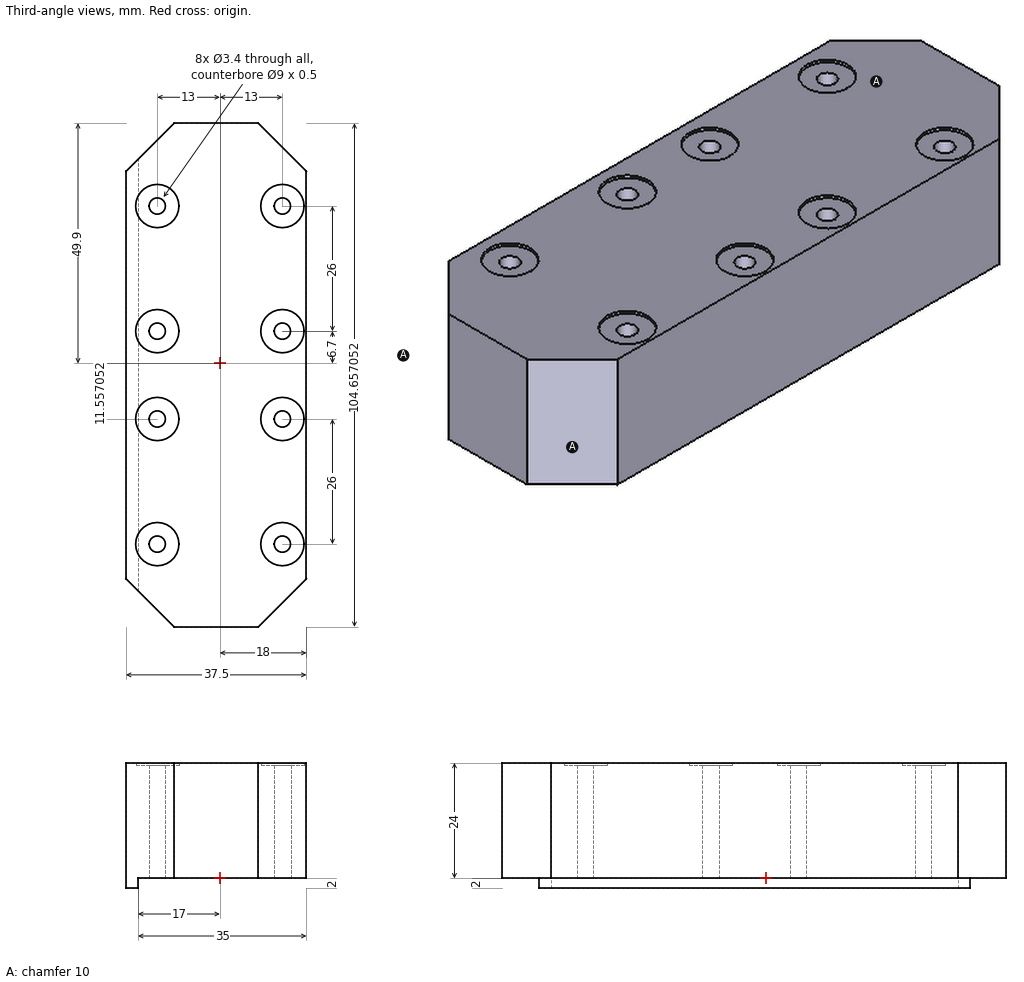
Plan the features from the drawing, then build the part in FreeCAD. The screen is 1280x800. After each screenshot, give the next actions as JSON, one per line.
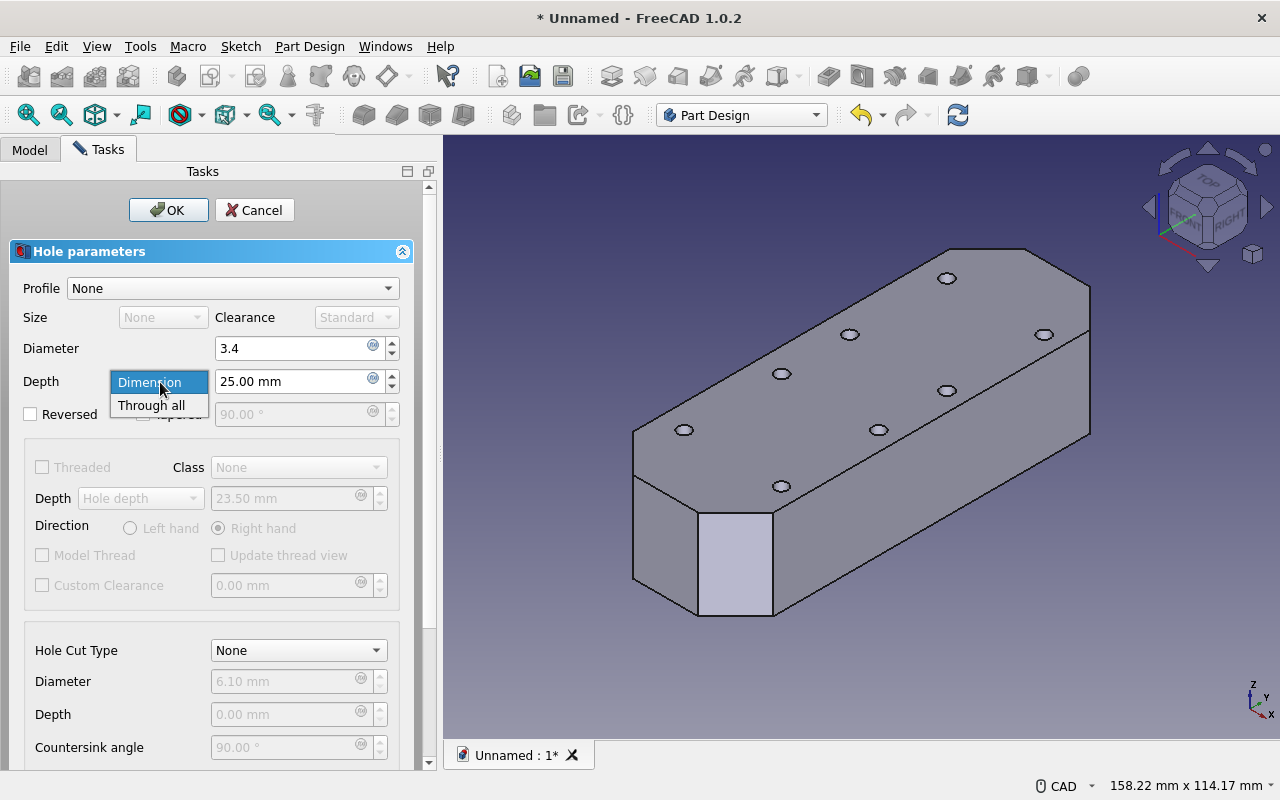
{"action": "left_click", "coordinate": [158, 406]}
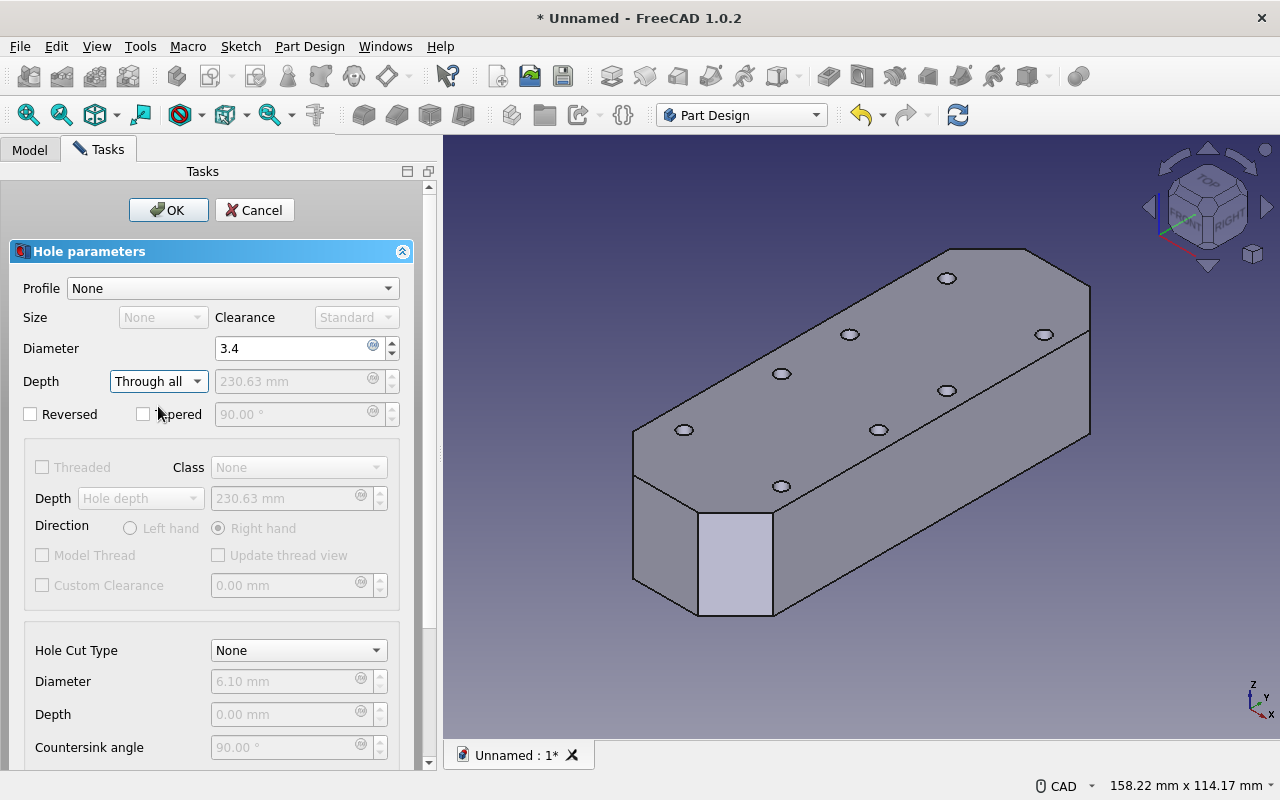
{"action": "left_click", "coordinate": [300, 650]}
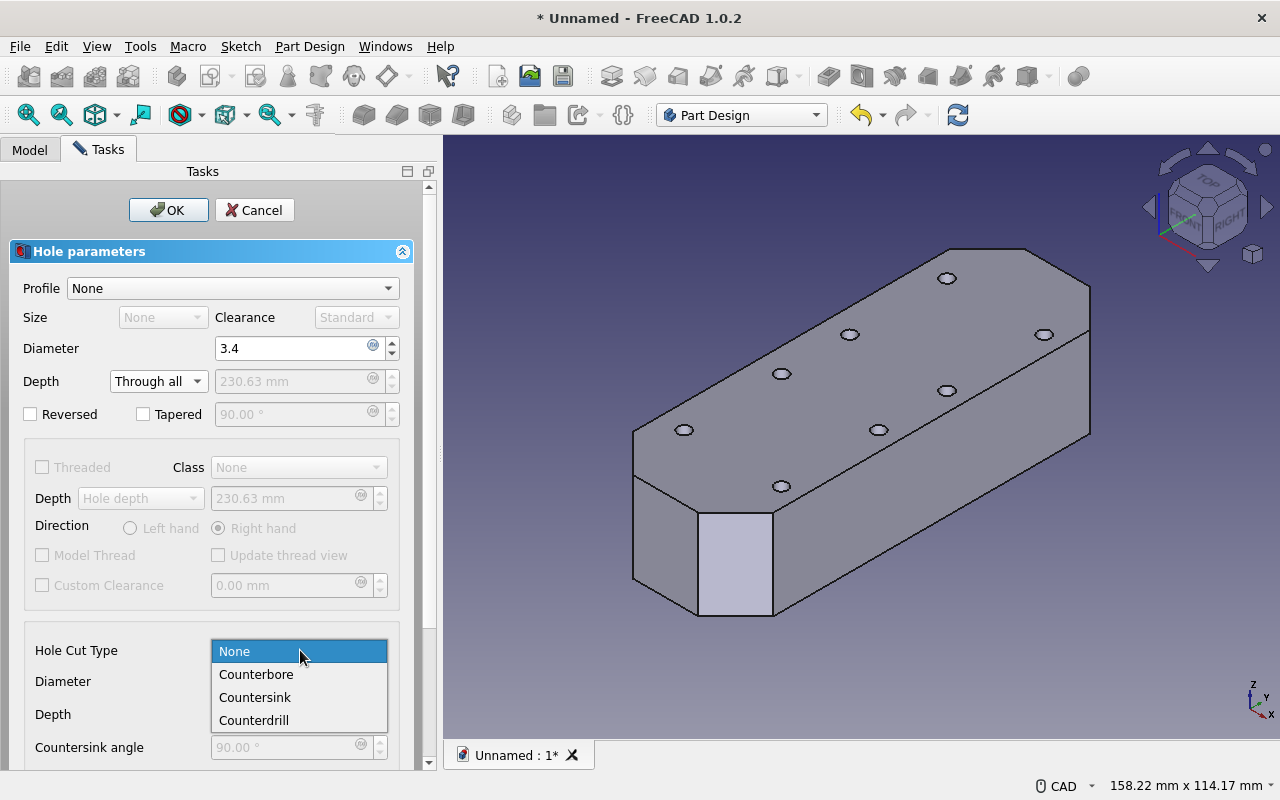
{"action": "left_click", "coordinate": [298, 674]}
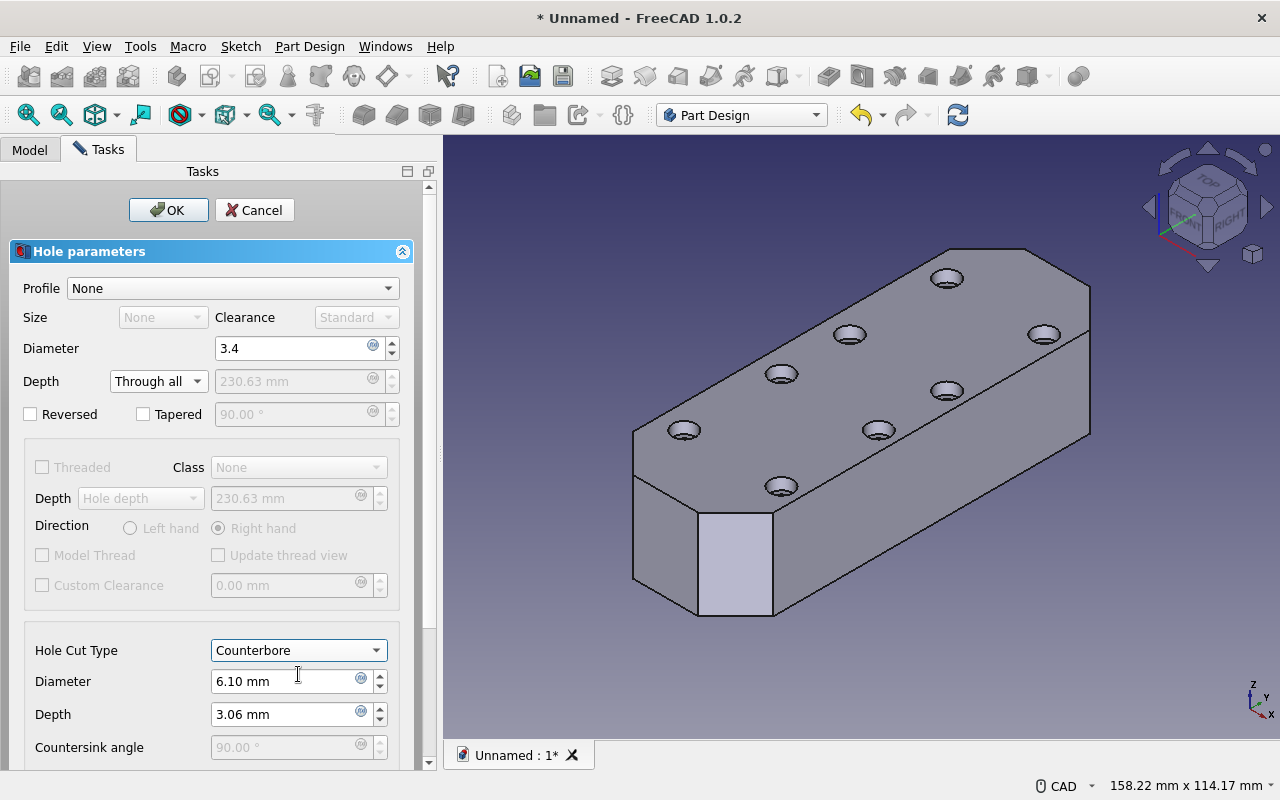
{"action": "triple_click", "coordinate": [292, 682]}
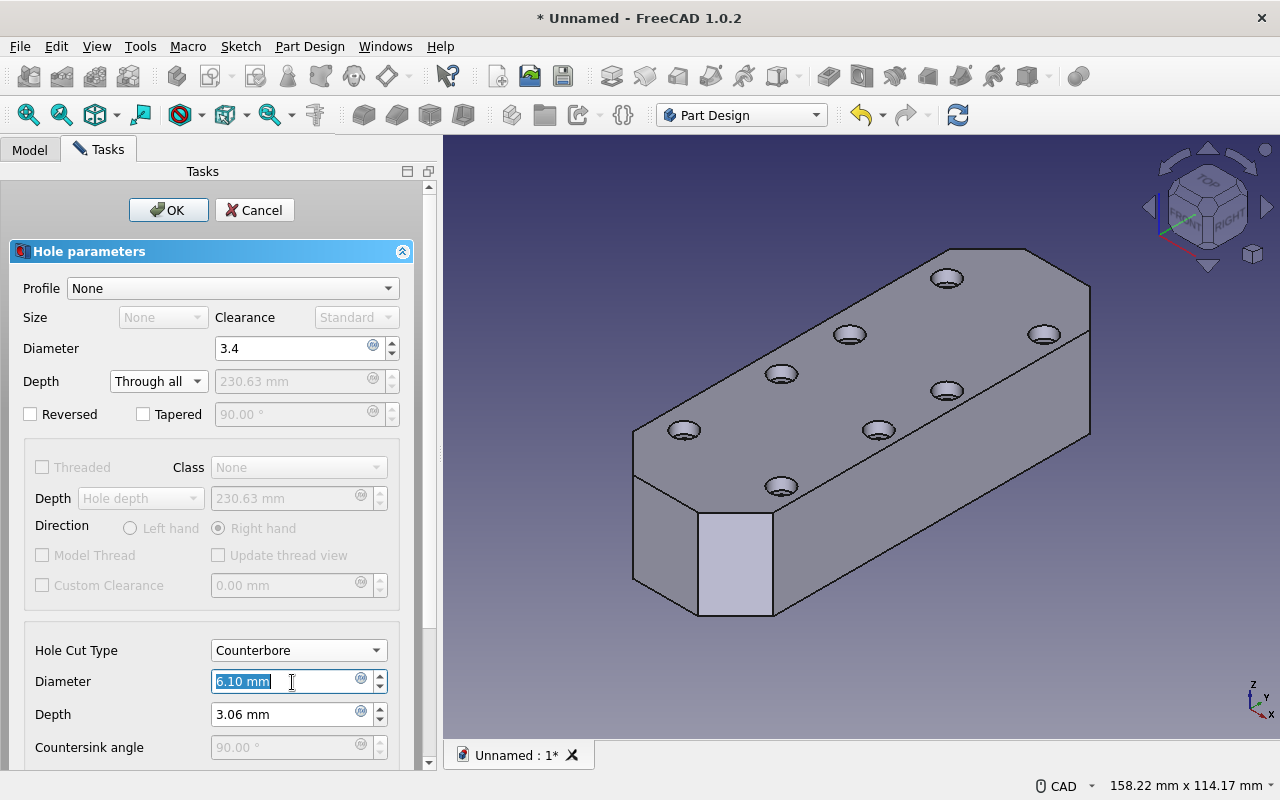
{"action": "type", "text": "9"}
{"action": "key", "text": "Tab"}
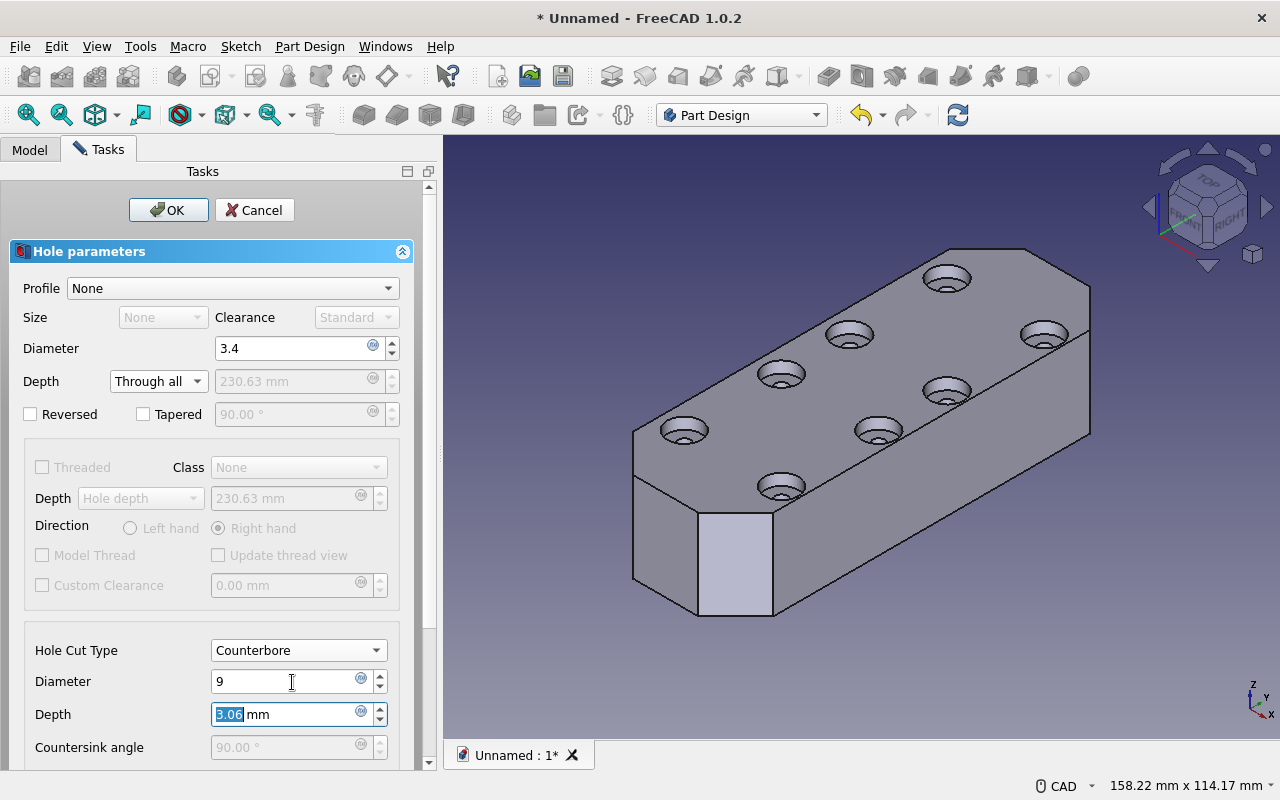
{"action": "type", "text": "0.5"}
{"action": "key", "text": "Tab"}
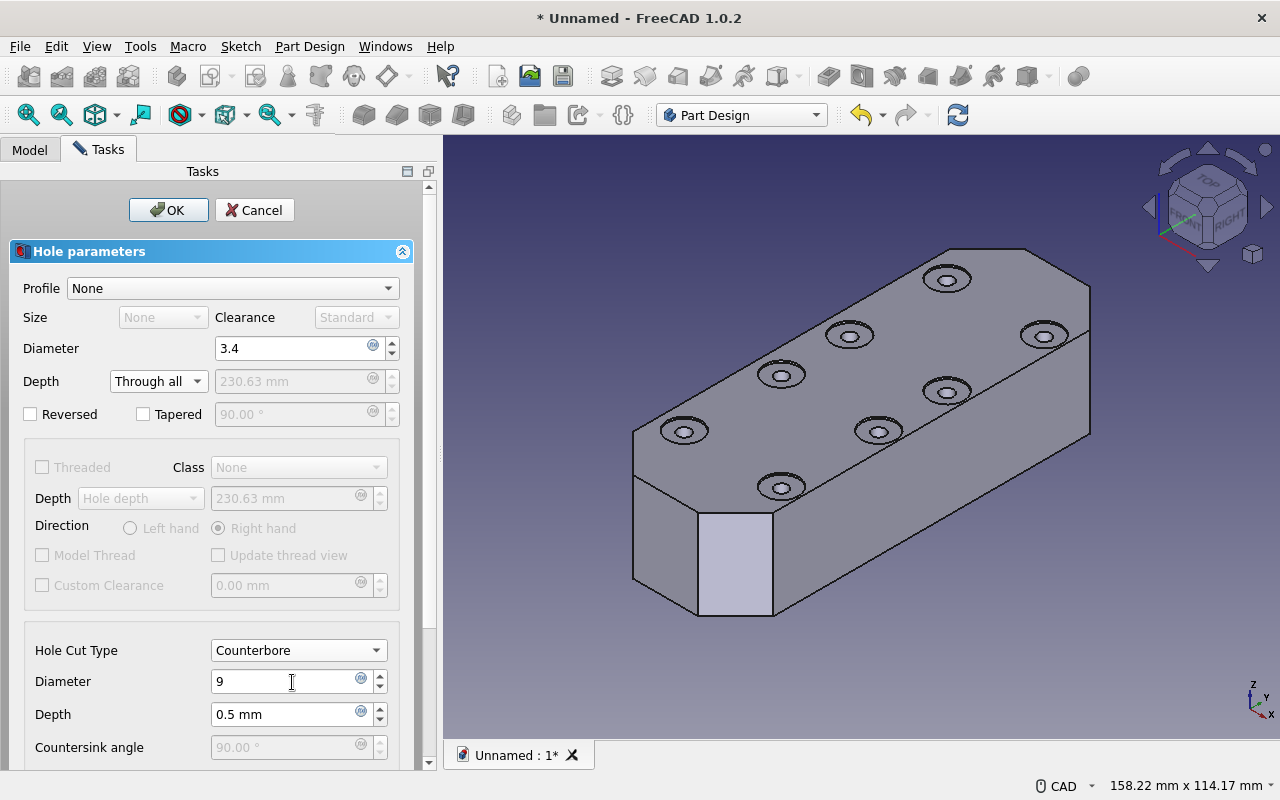
{"action": "left_click", "coordinate": [169, 210]}